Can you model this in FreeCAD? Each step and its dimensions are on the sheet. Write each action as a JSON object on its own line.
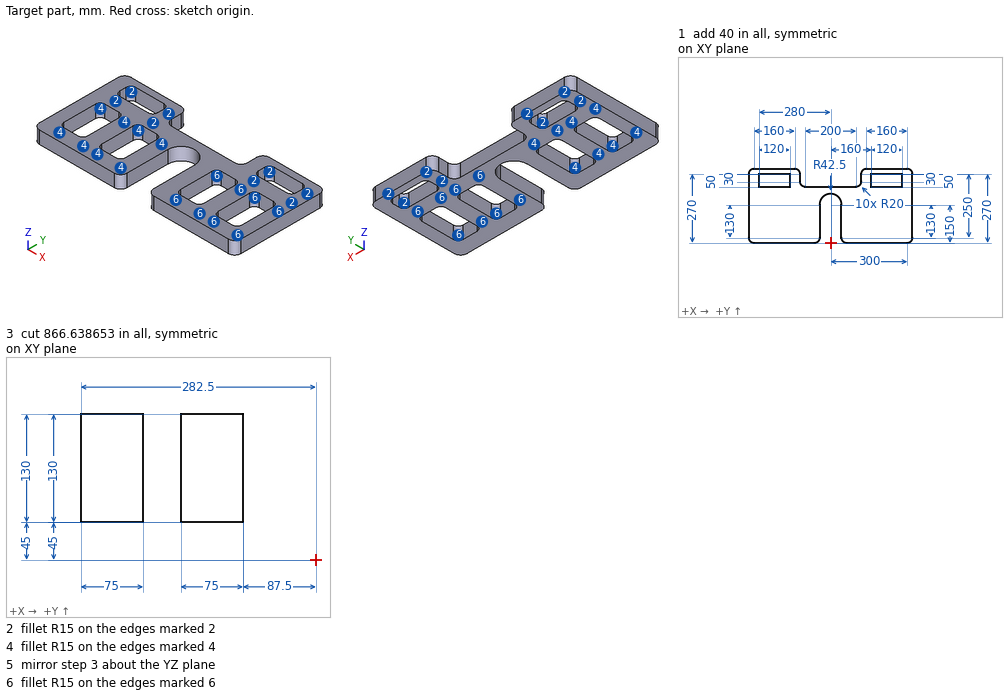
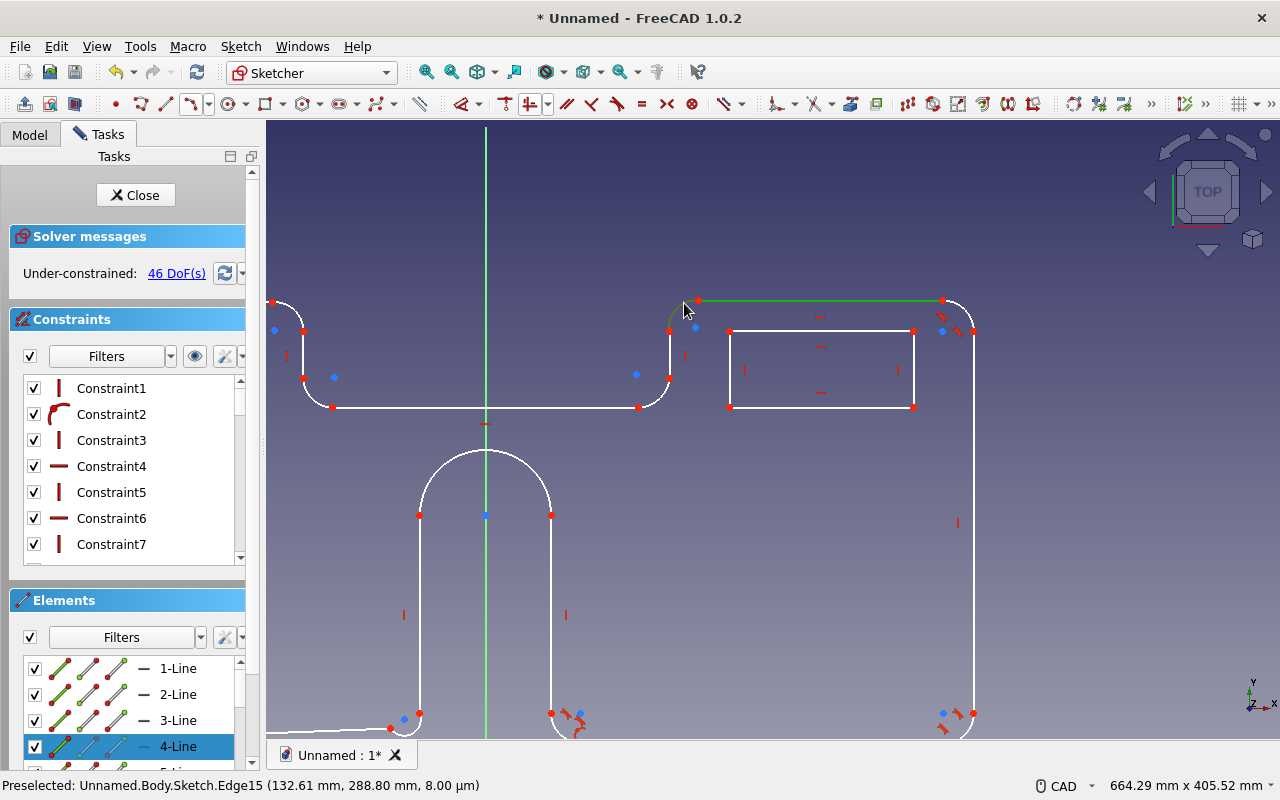
{"action": "key", "text": "t"}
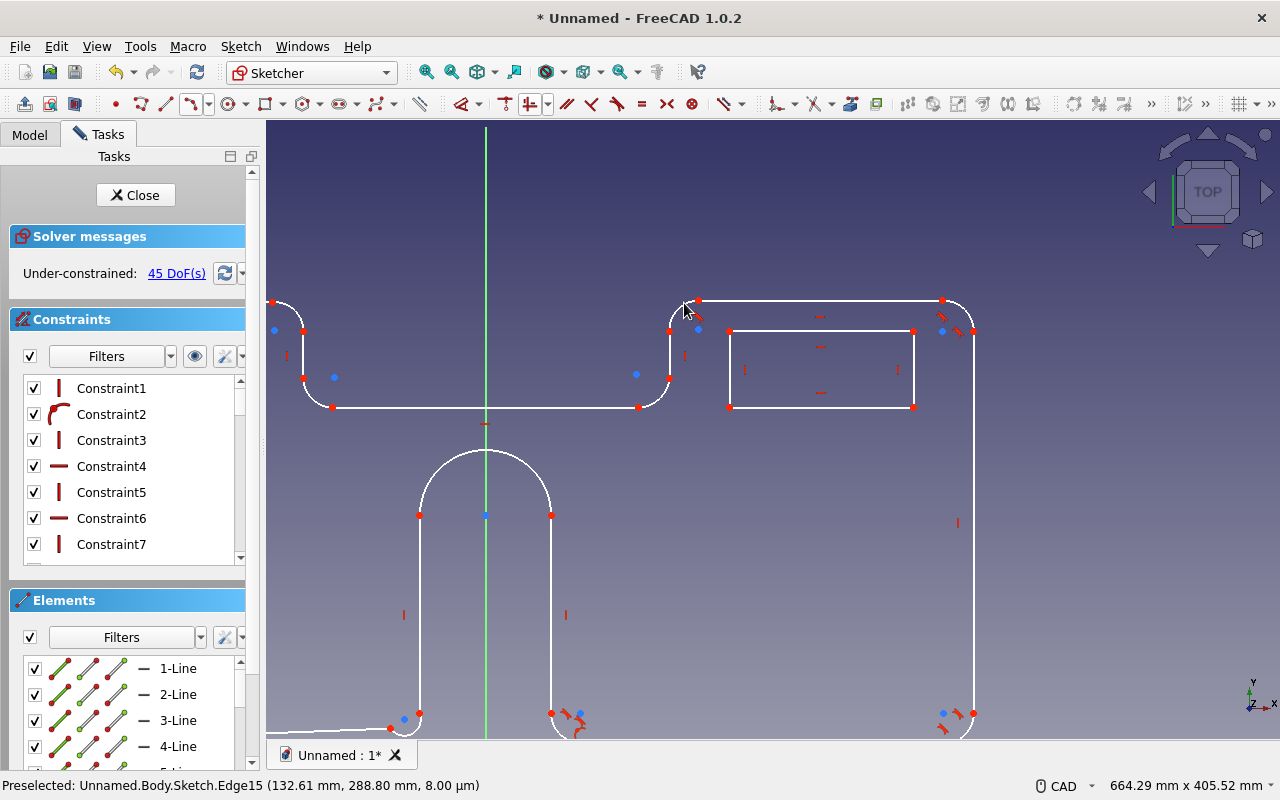
{"action": "left_click", "coordinate": [670, 346]}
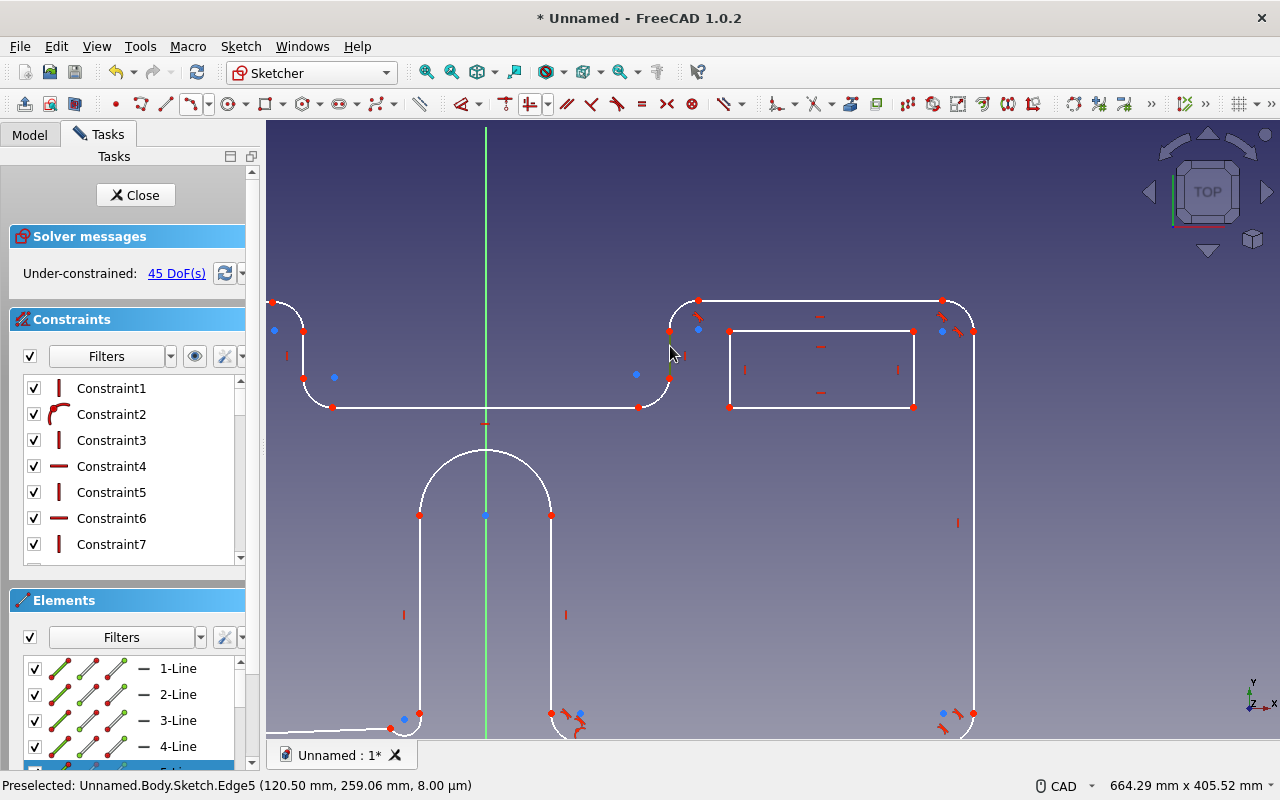
{"action": "left_click", "coordinate": [685, 304]}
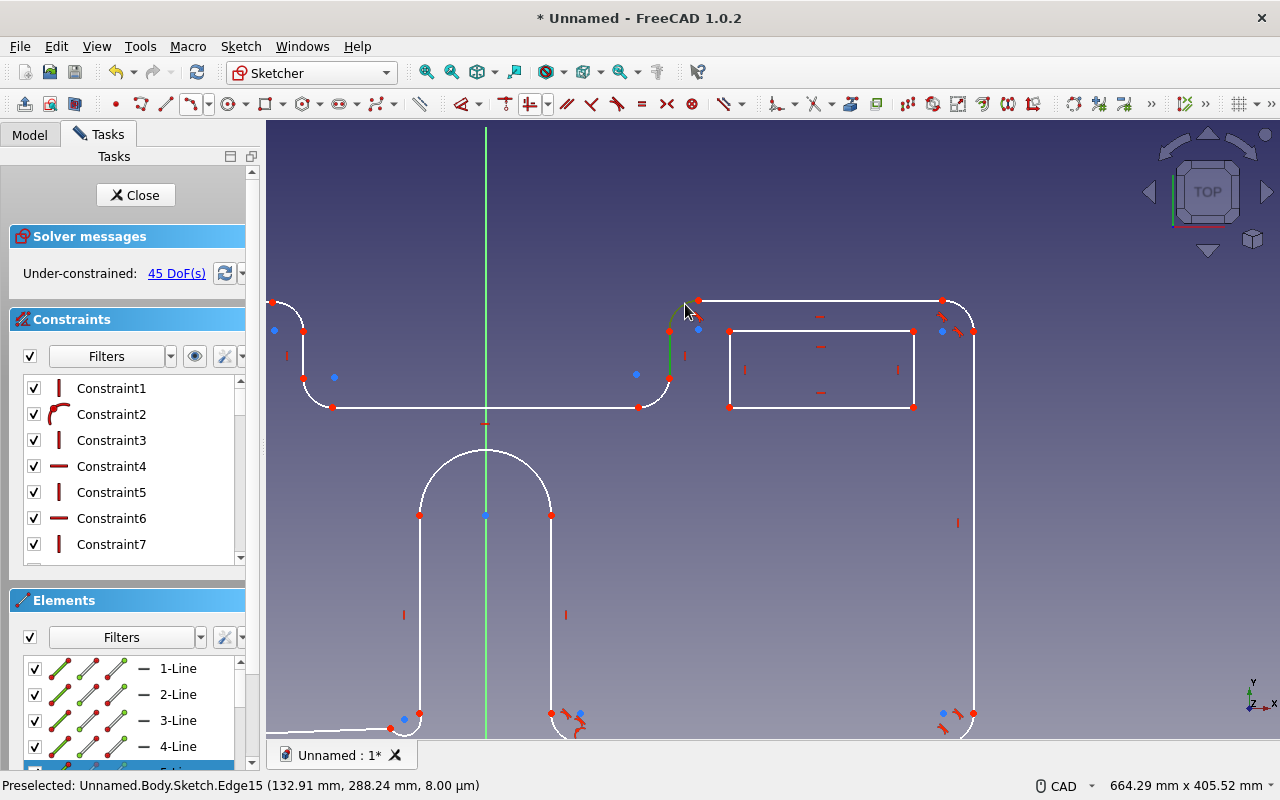
{"action": "left_click", "coordinate": [617, 104]}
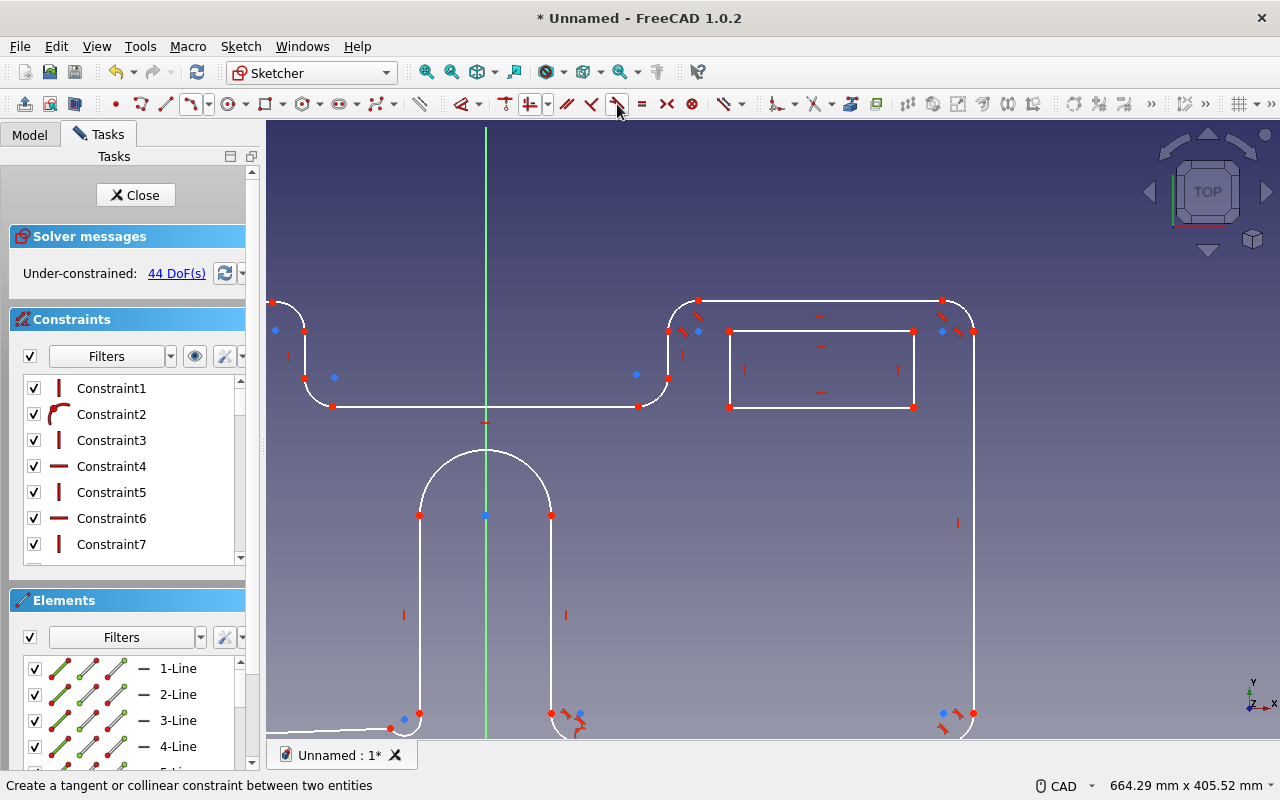
{"action": "left_click", "coordinate": [668, 346]}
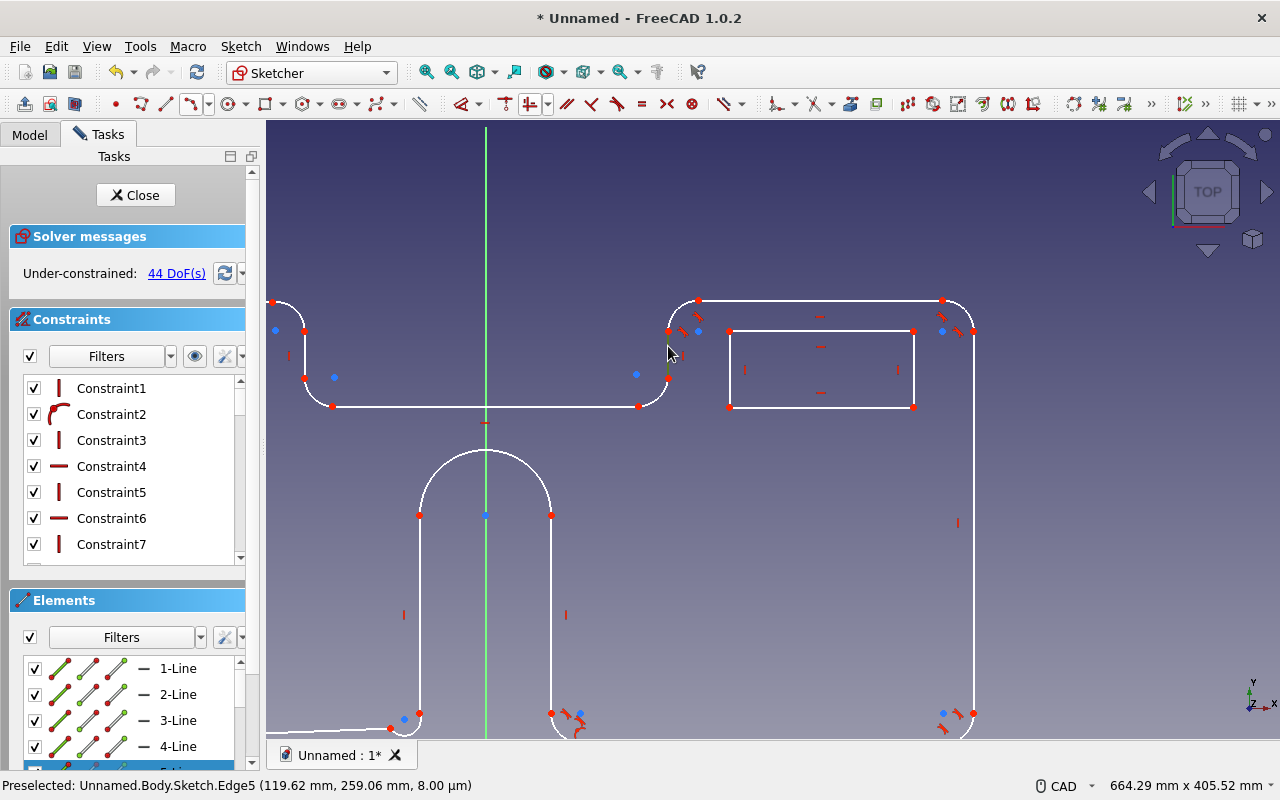
{"action": "left_click", "coordinate": [651, 403]}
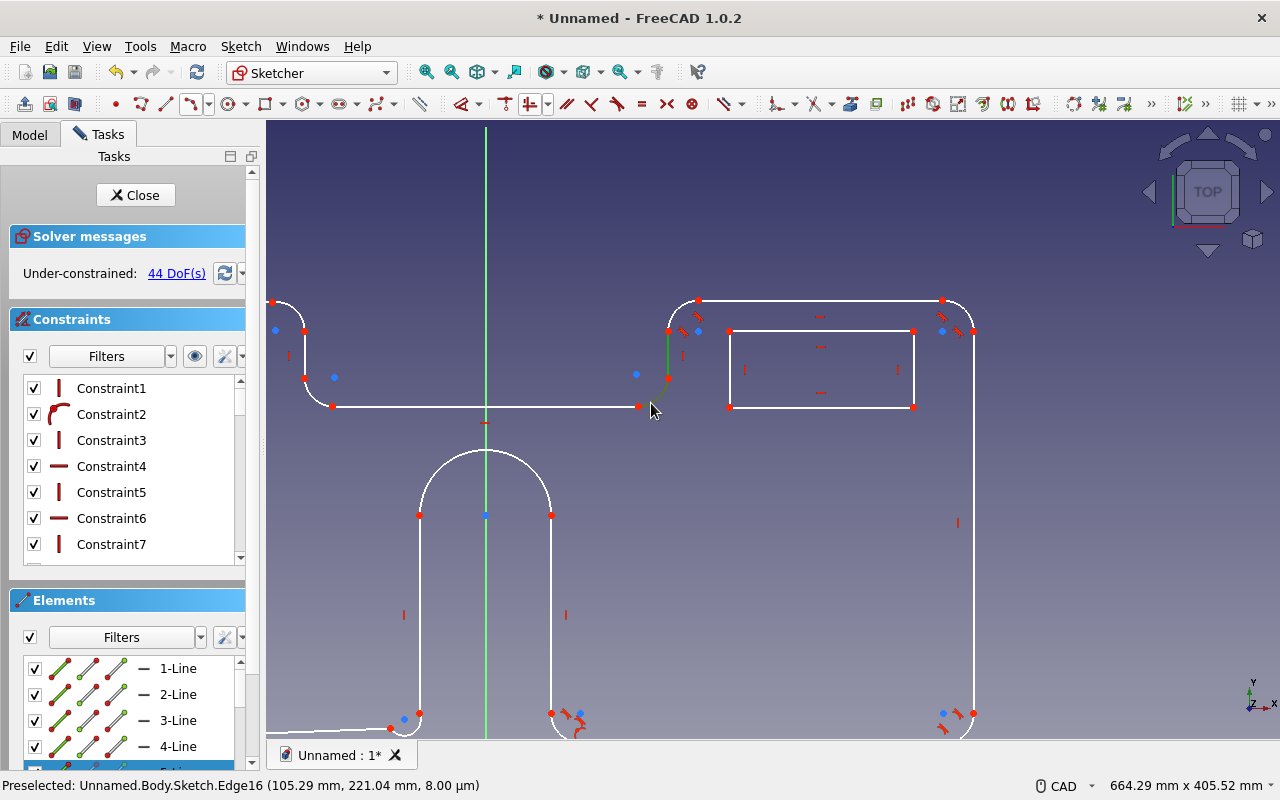
{"action": "left_click", "coordinate": [617, 104]}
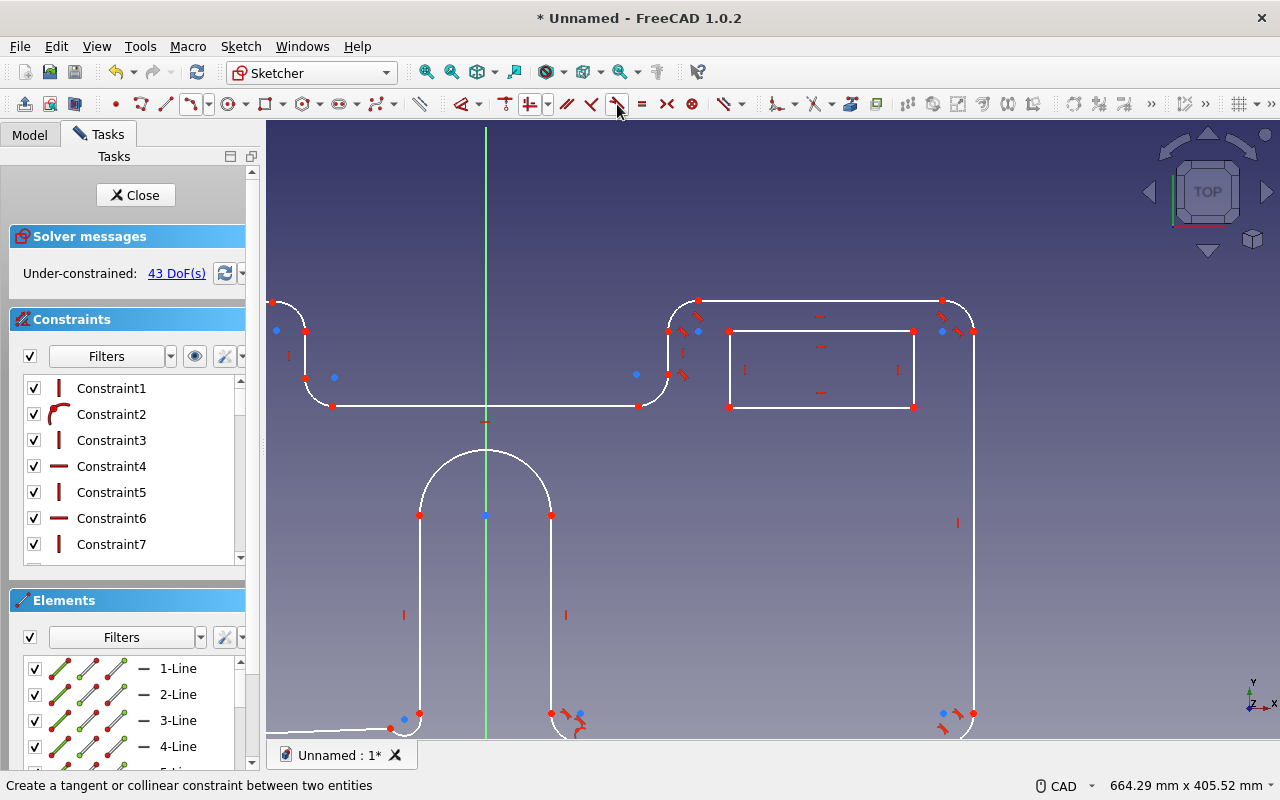
{"action": "left_click", "coordinate": [547, 406]}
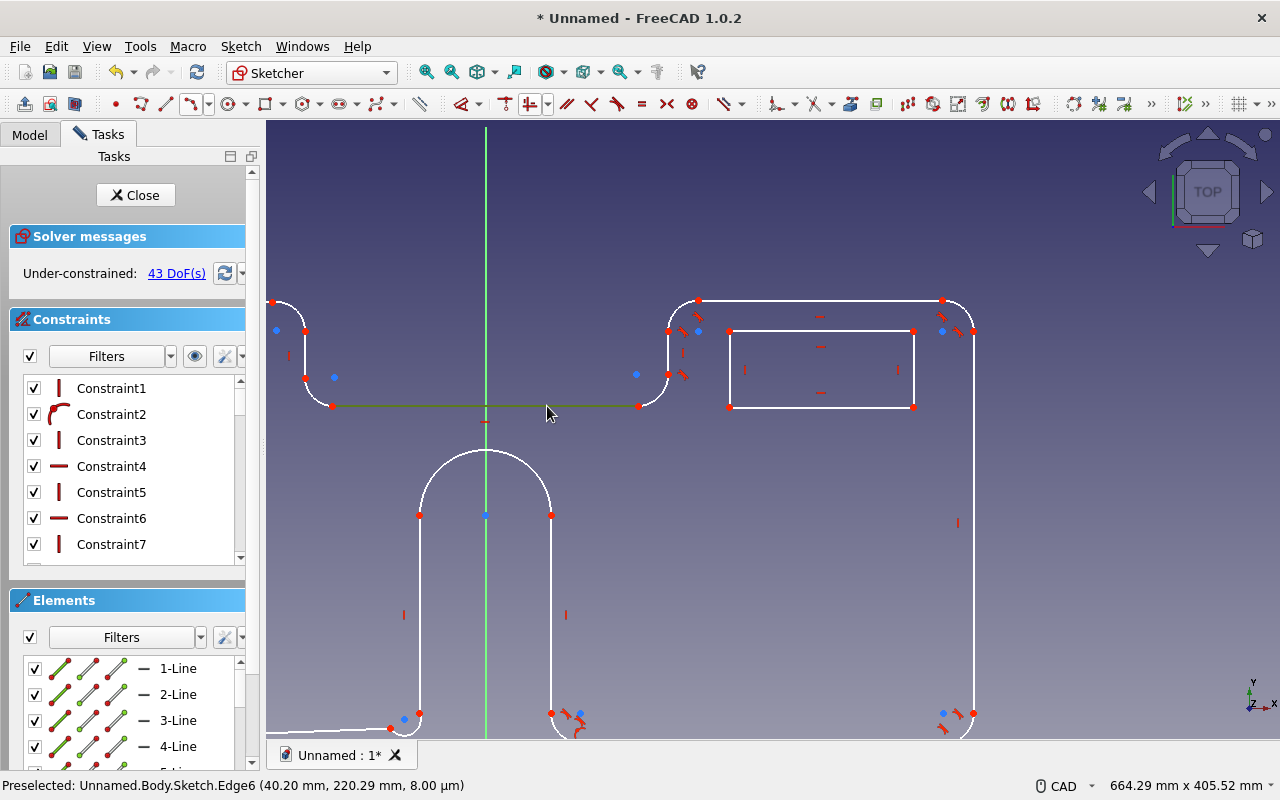
{"action": "left_click", "coordinate": [652, 402]}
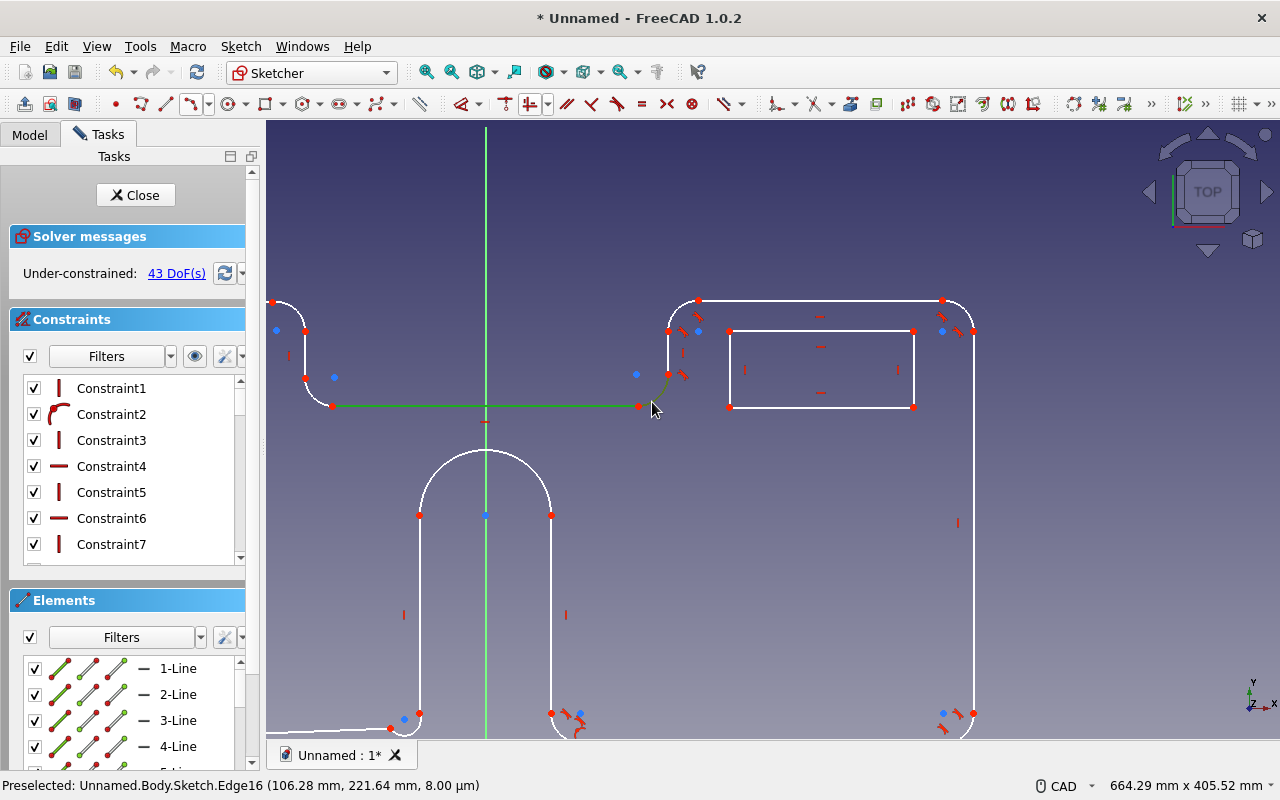
{"action": "left_click", "coordinate": [617, 104]}